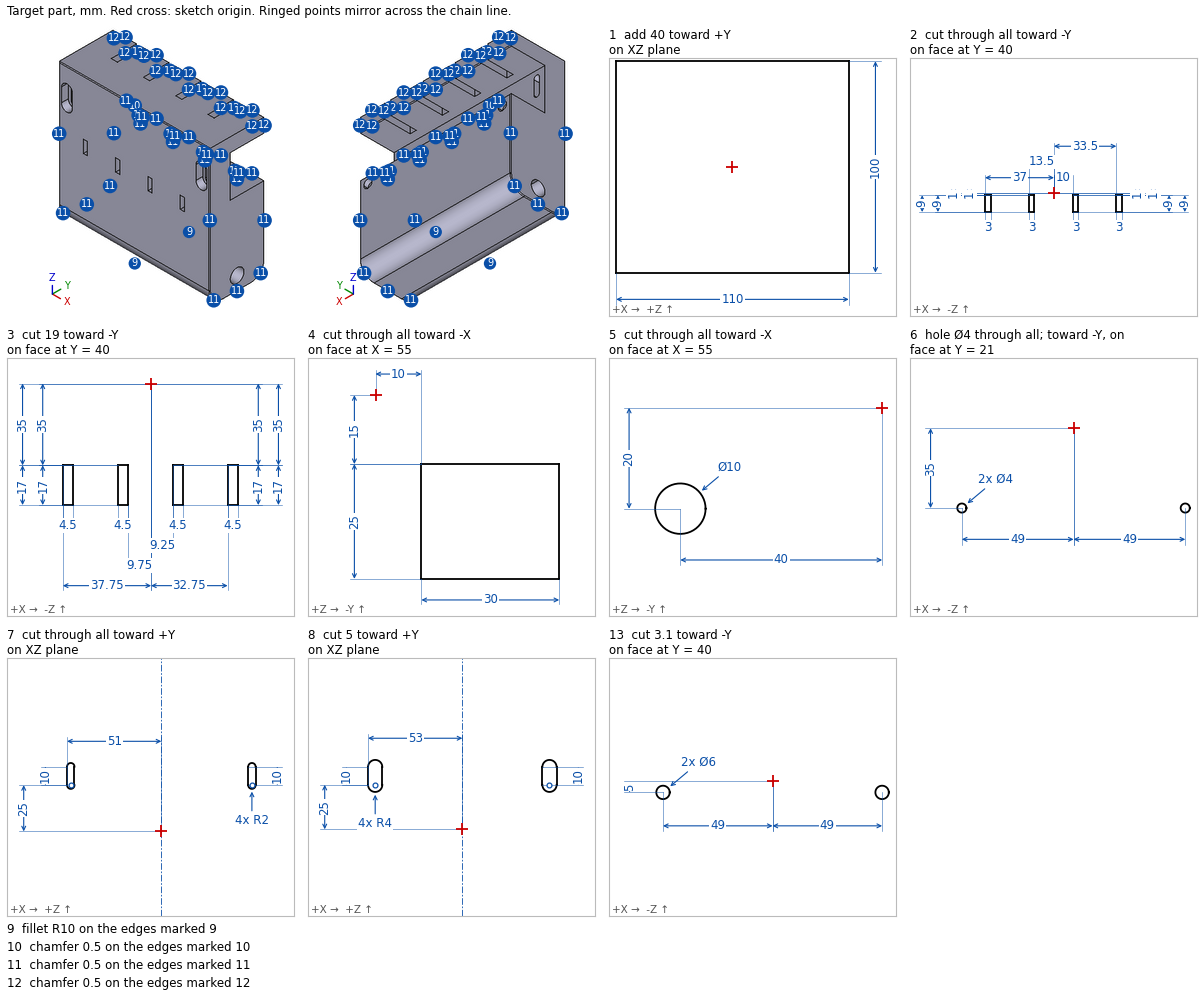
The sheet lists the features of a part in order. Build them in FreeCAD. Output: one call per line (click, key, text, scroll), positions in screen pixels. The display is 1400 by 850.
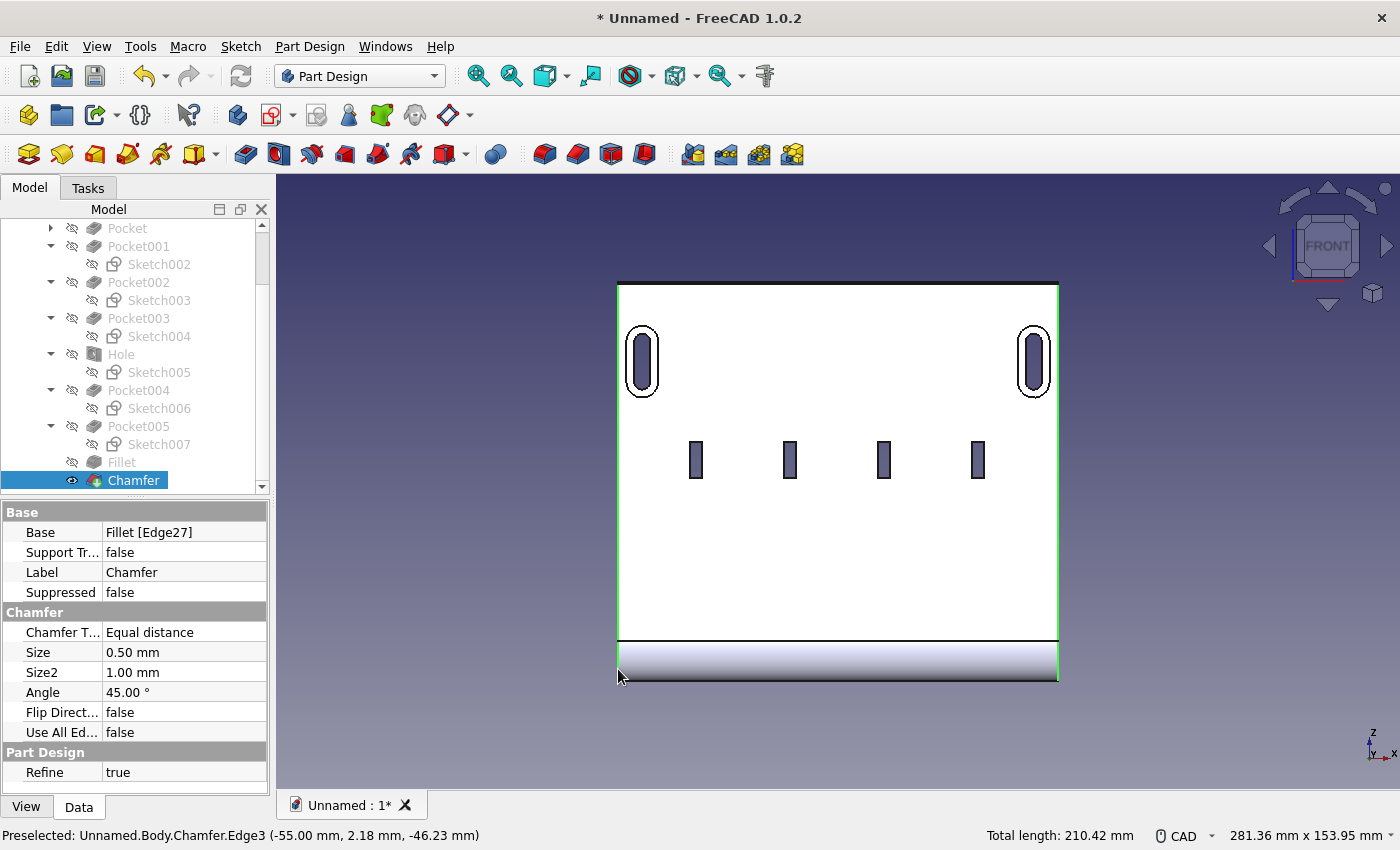
key(3)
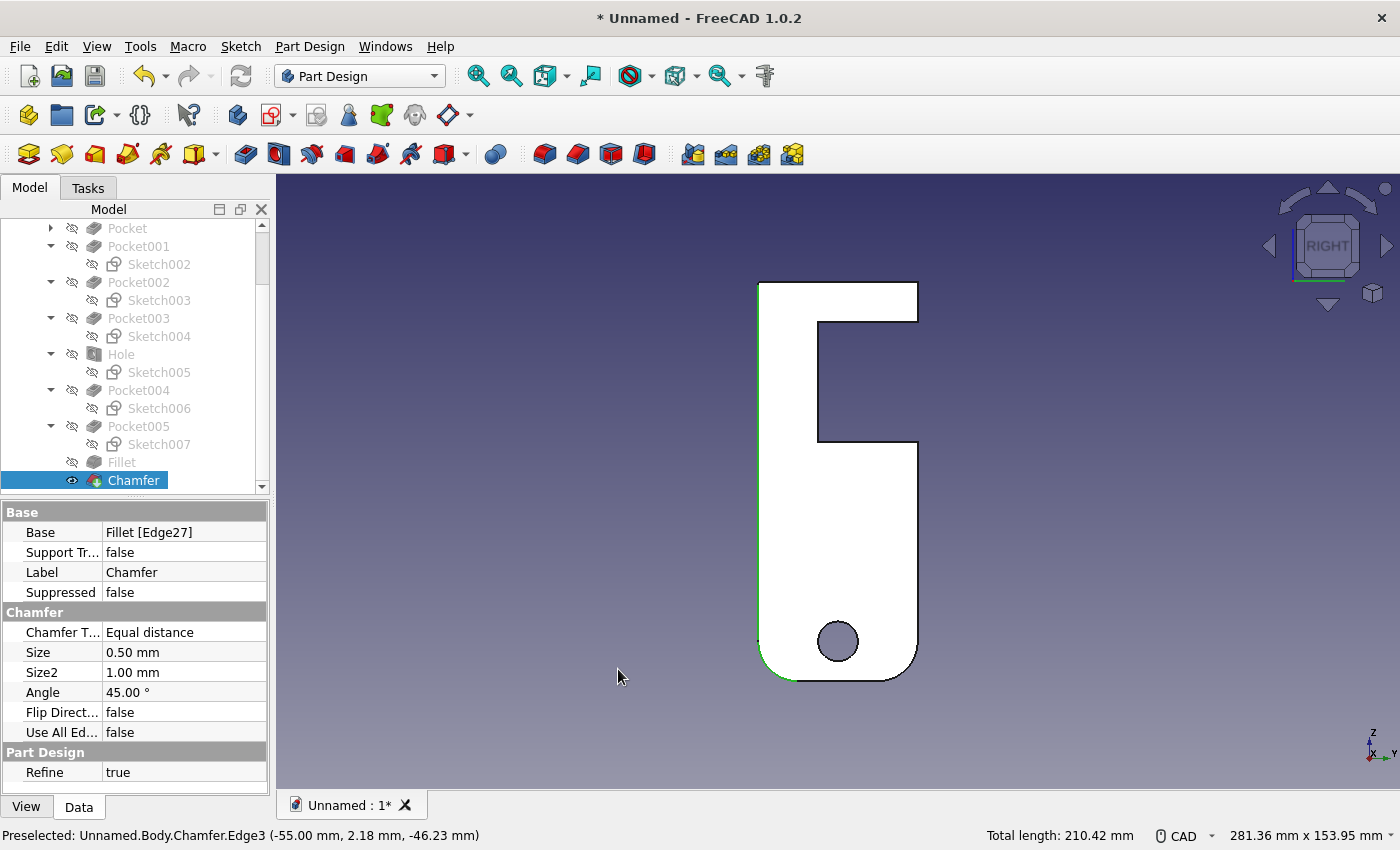
click(838, 680, ctrl)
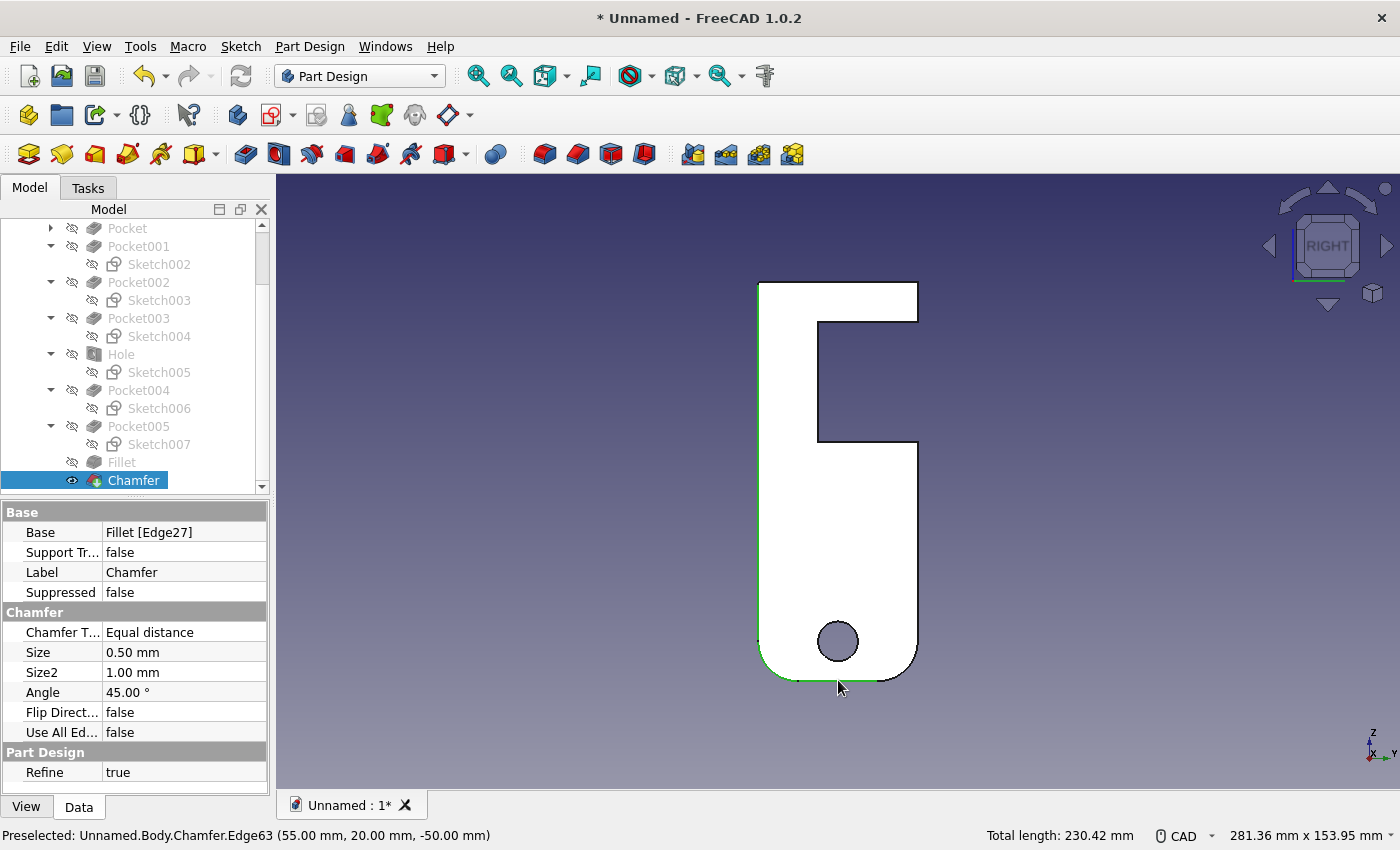
click(906, 669, ctrl)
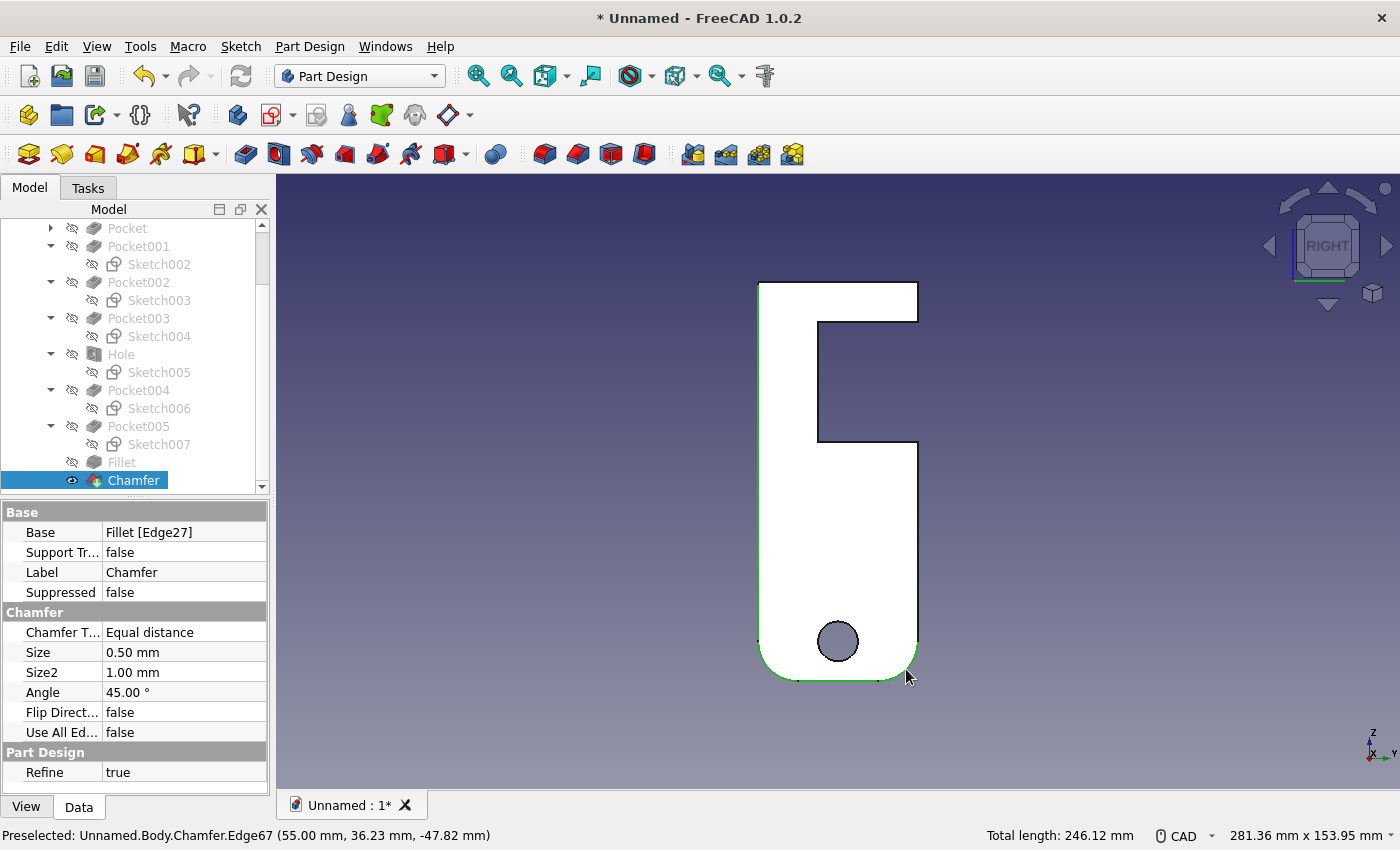
click(918, 540, ctrl)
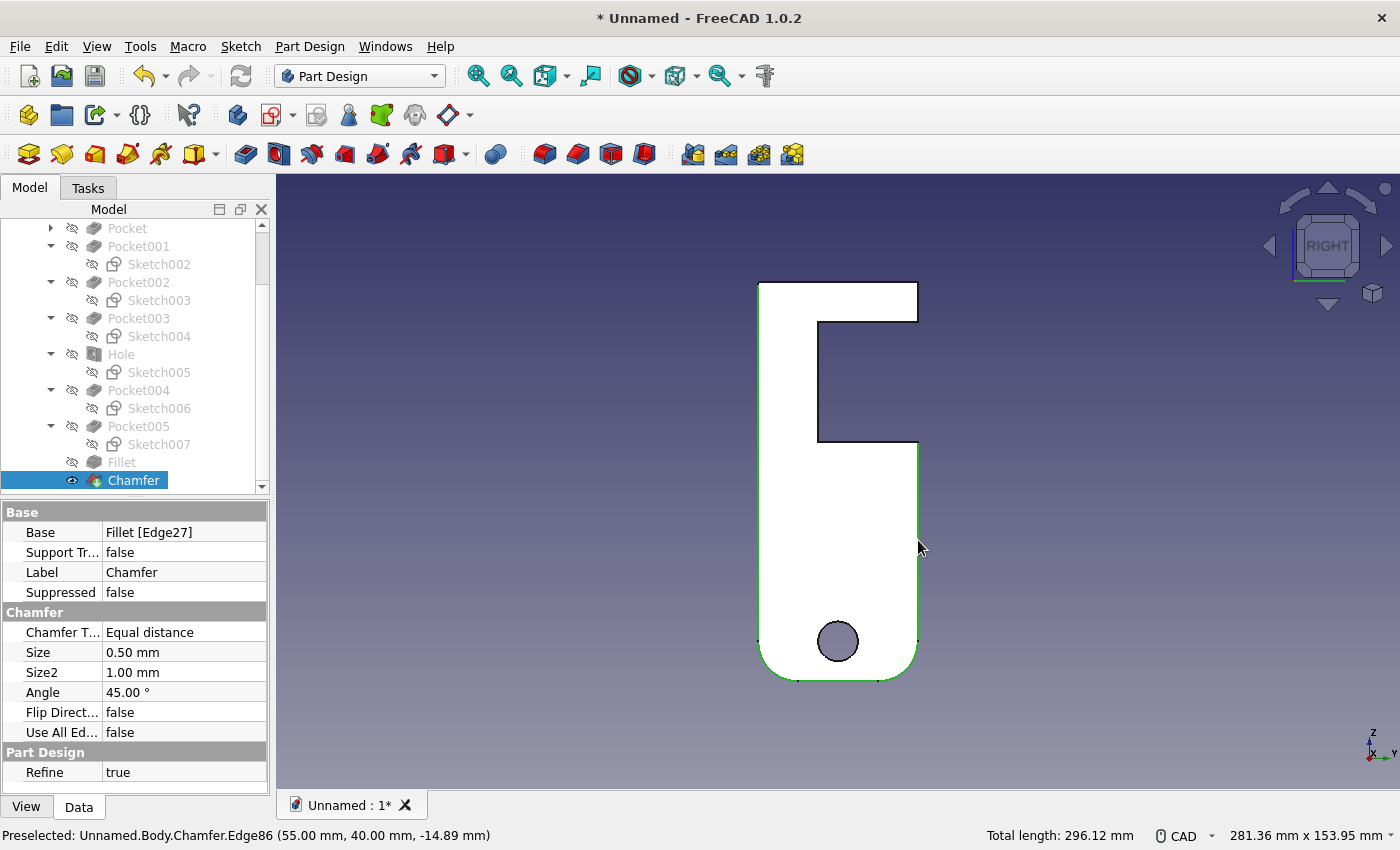
key(5)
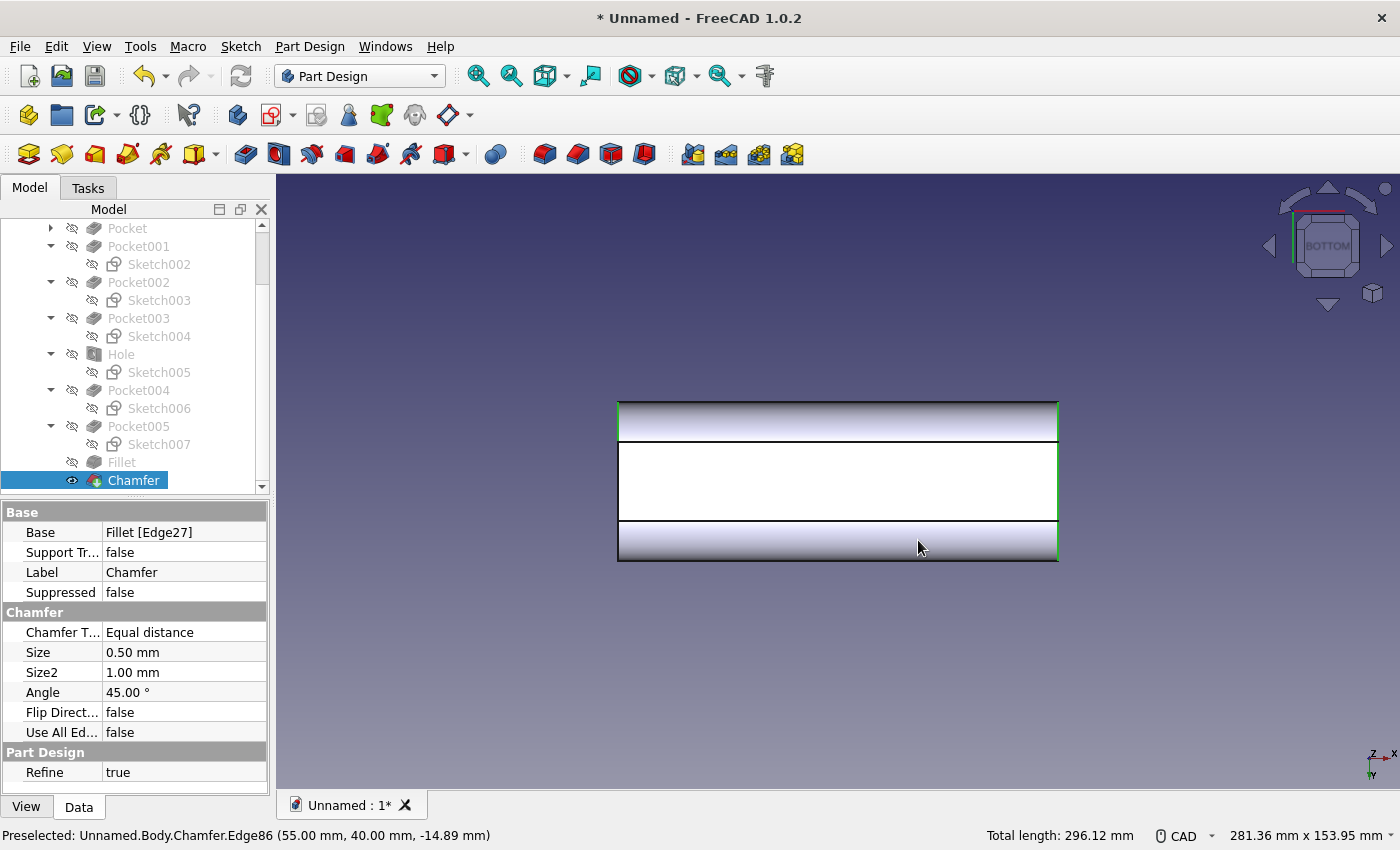
key(v)
key(f)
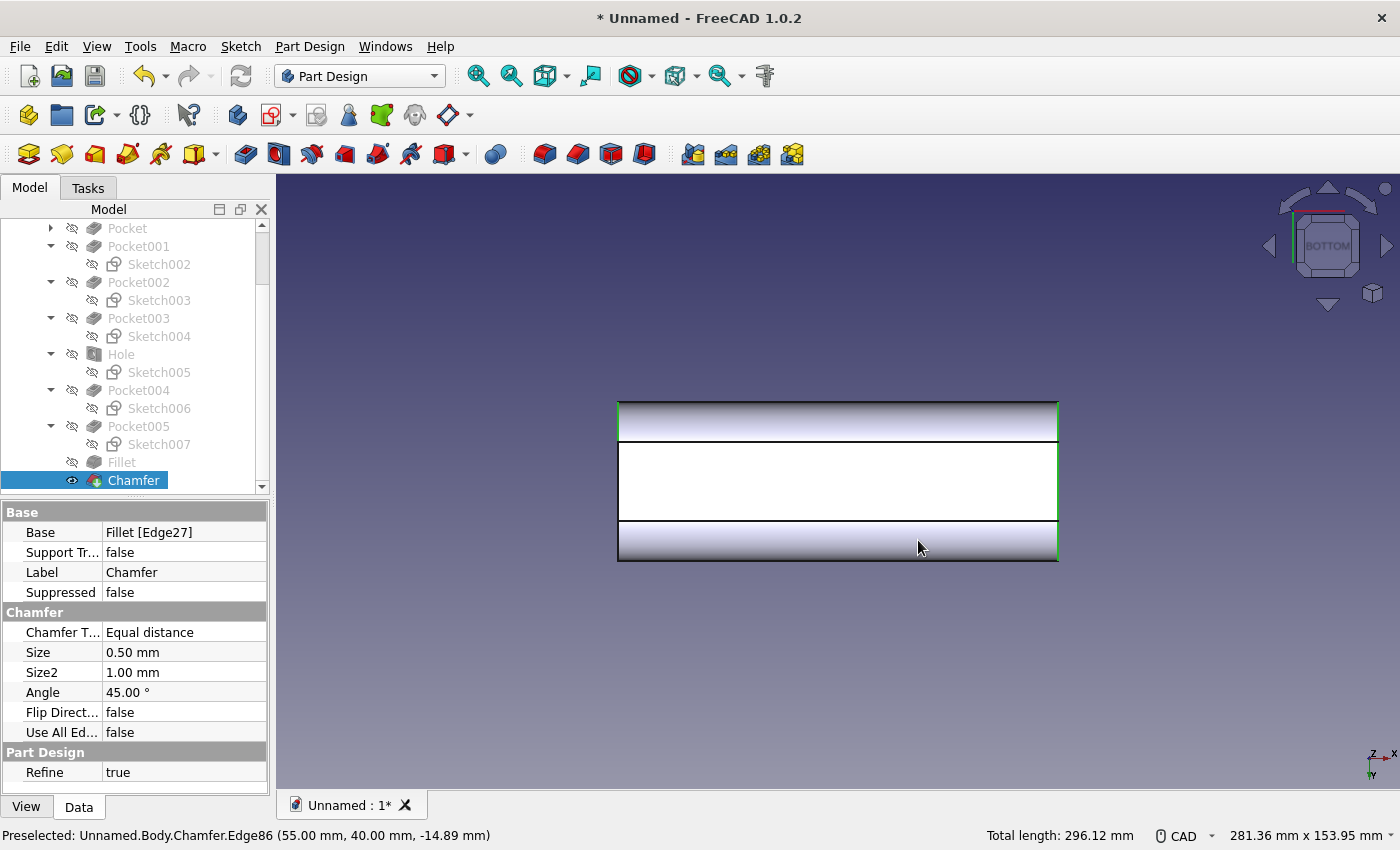
click(618, 480, ctrl)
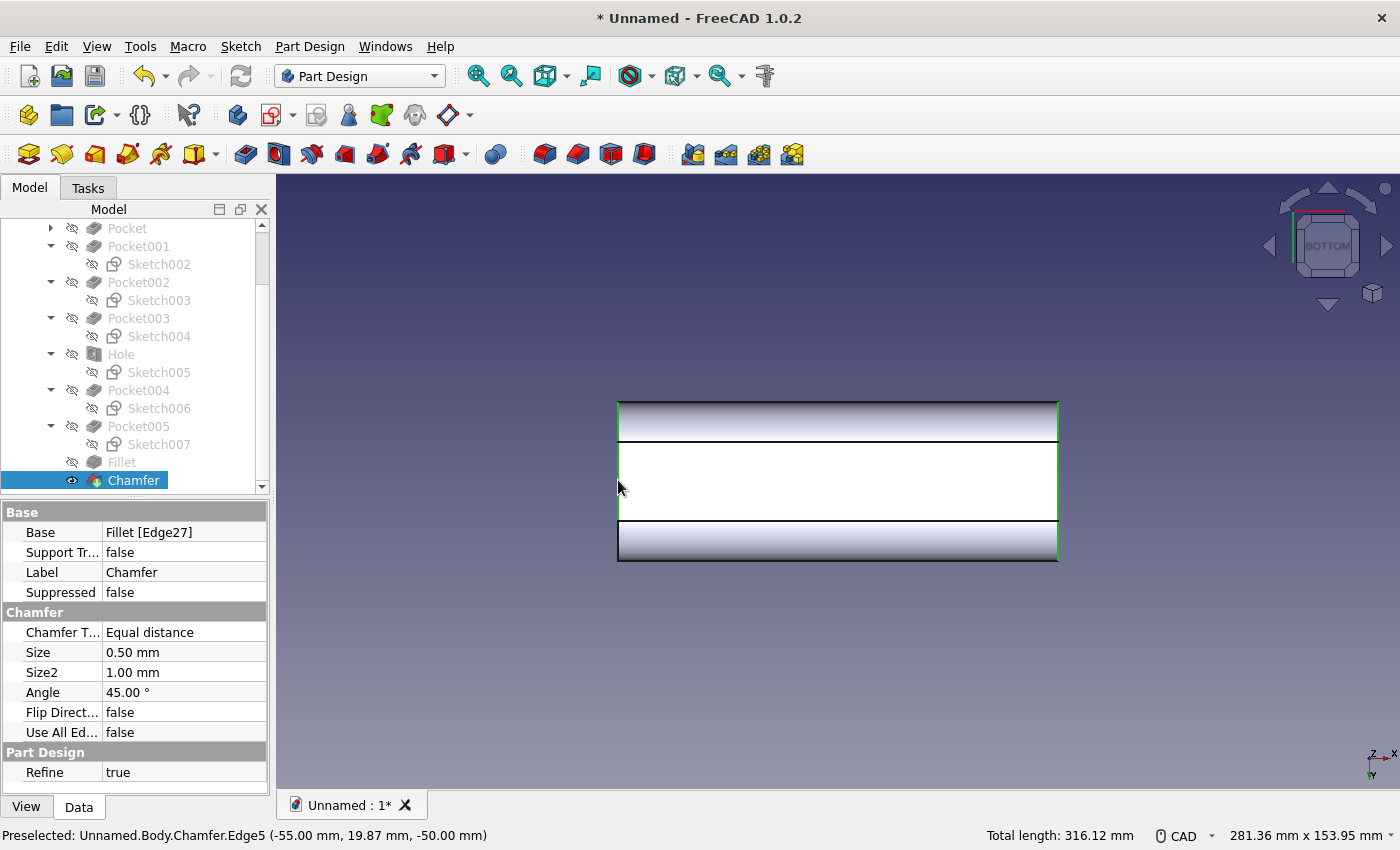
click(618, 549, ctrl)